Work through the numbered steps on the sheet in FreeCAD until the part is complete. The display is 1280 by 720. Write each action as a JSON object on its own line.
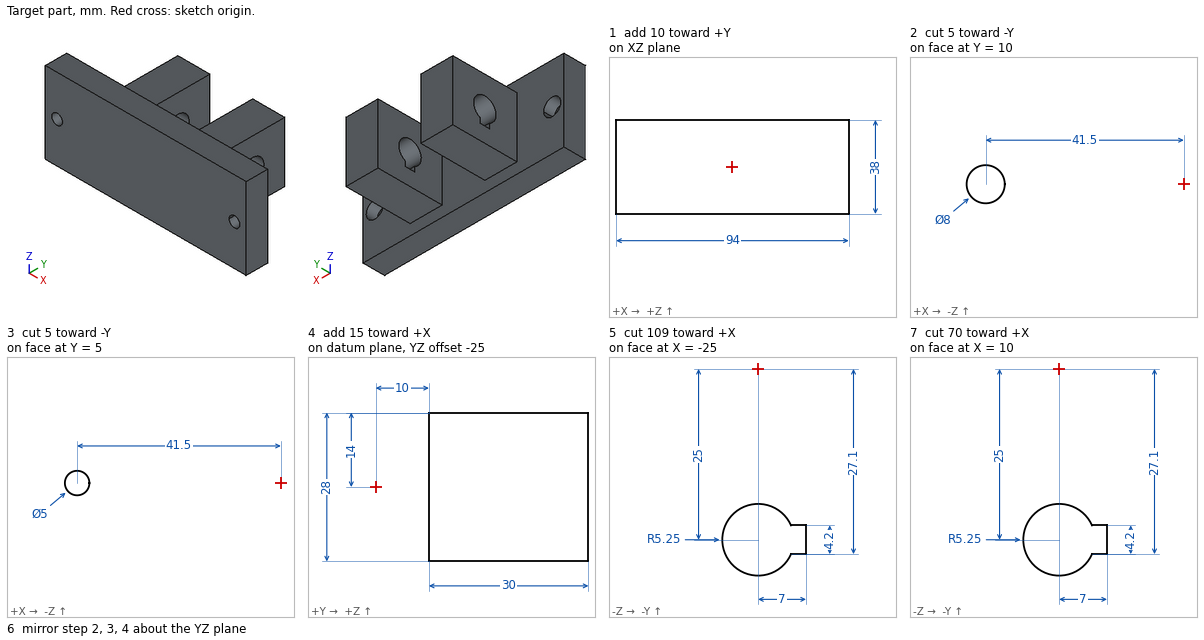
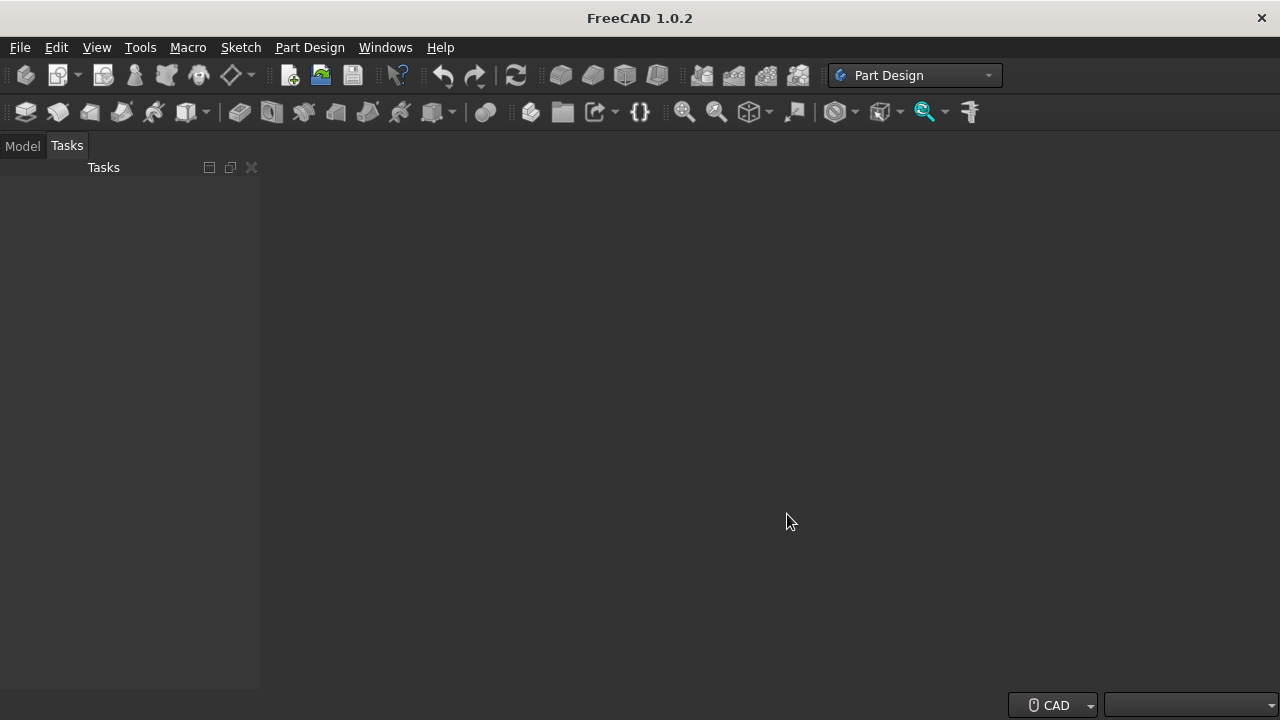
{"action": "left_click", "coordinate": [290, 76]}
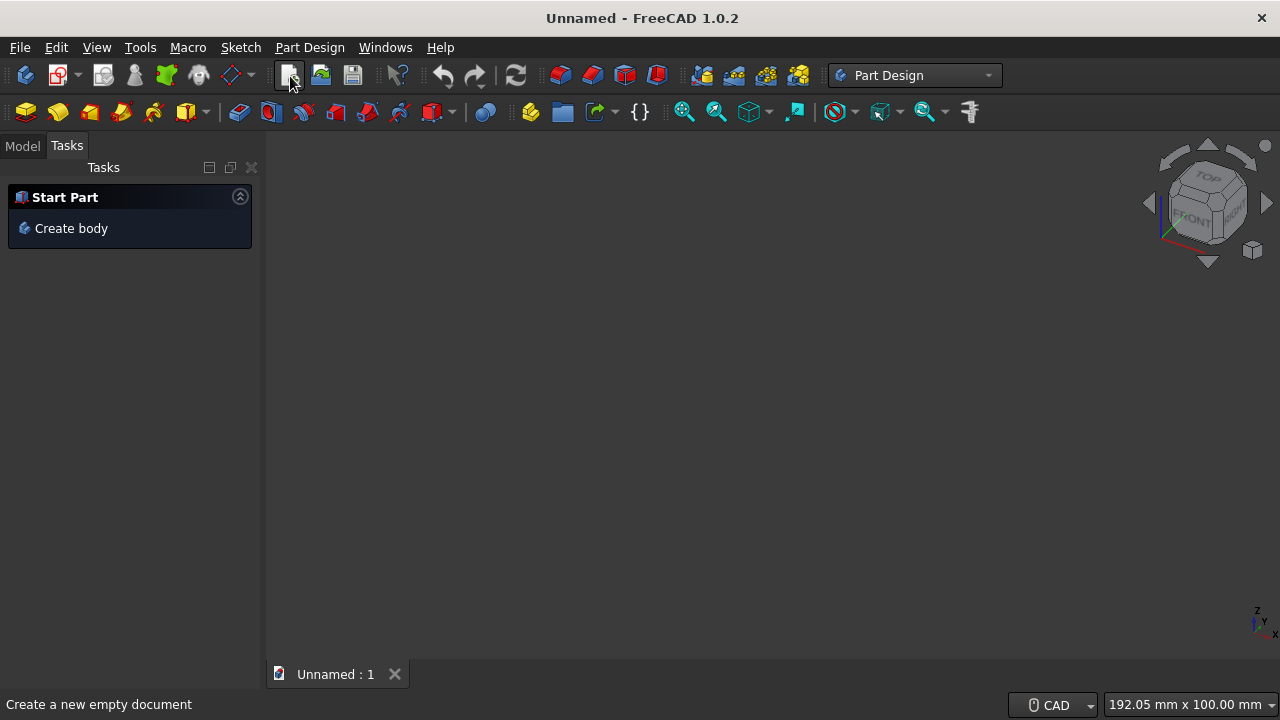
{"action": "left_click", "coordinate": [58, 76]}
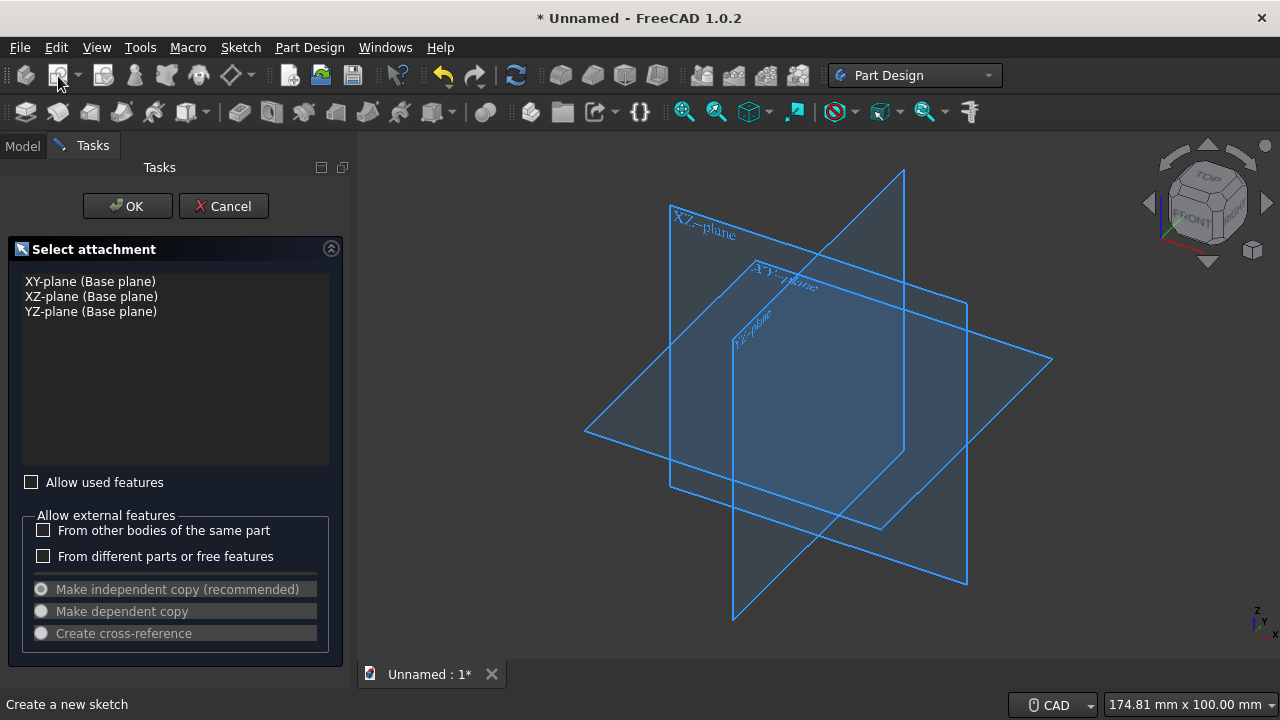
{"action": "left_click", "coordinate": [82, 296]}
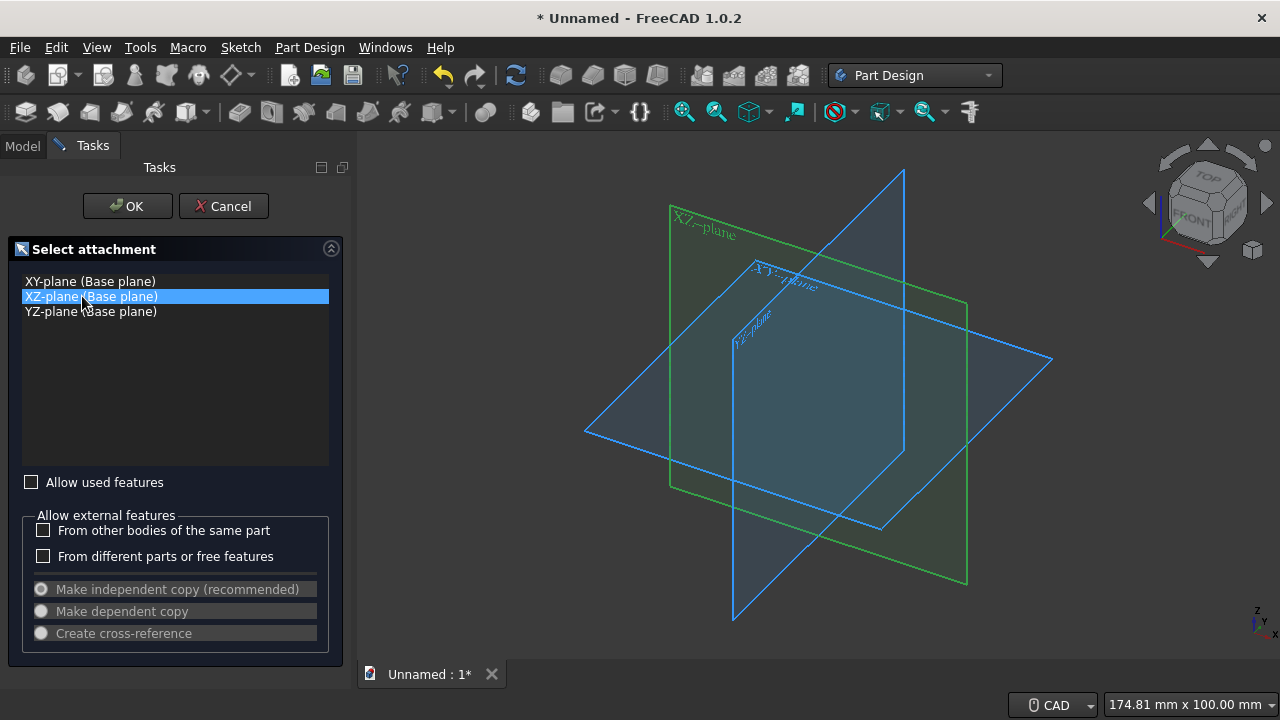
{"action": "left_click", "coordinate": [128, 206]}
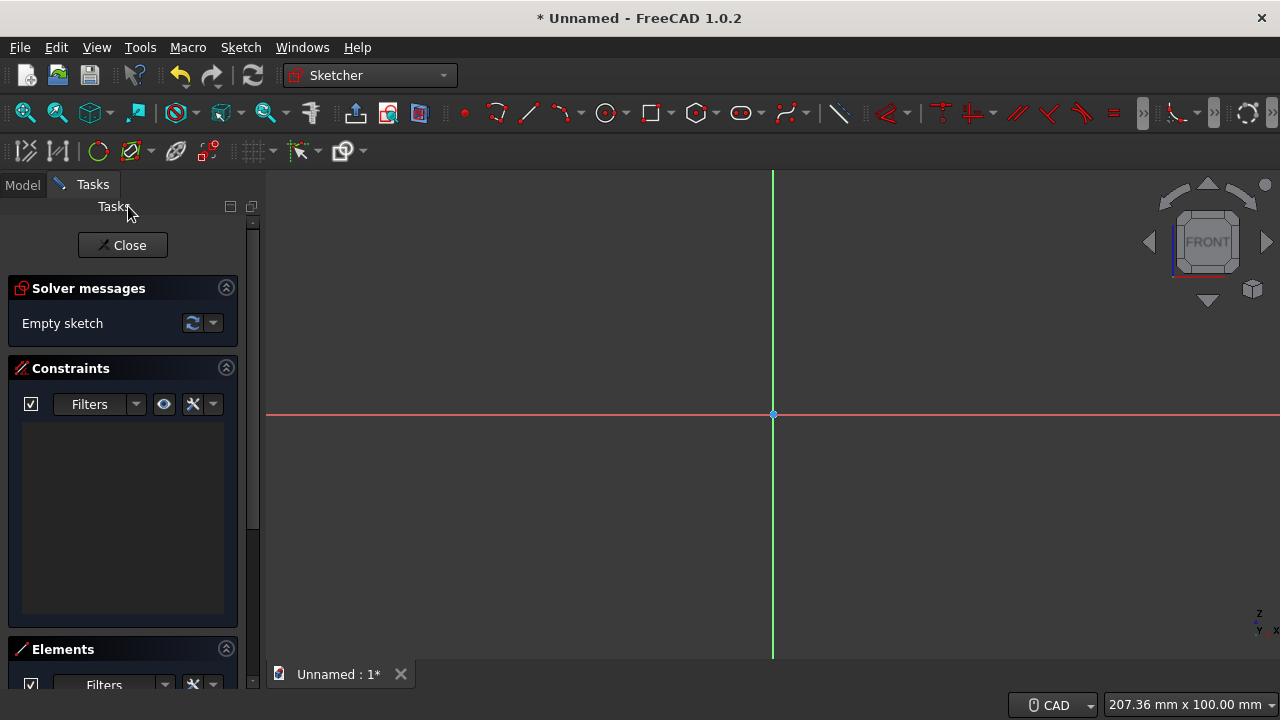
{"action": "left_click", "coordinate": [674, 114]}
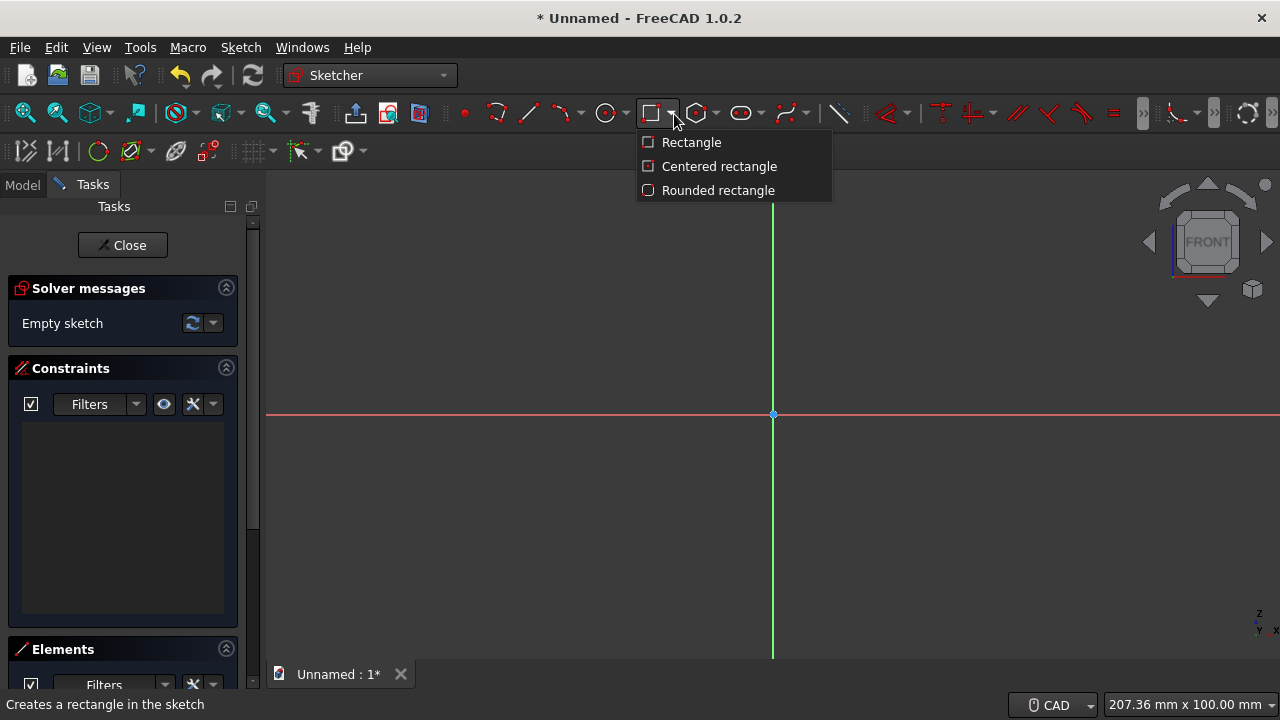
{"action": "left_click", "coordinate": [734, 166]}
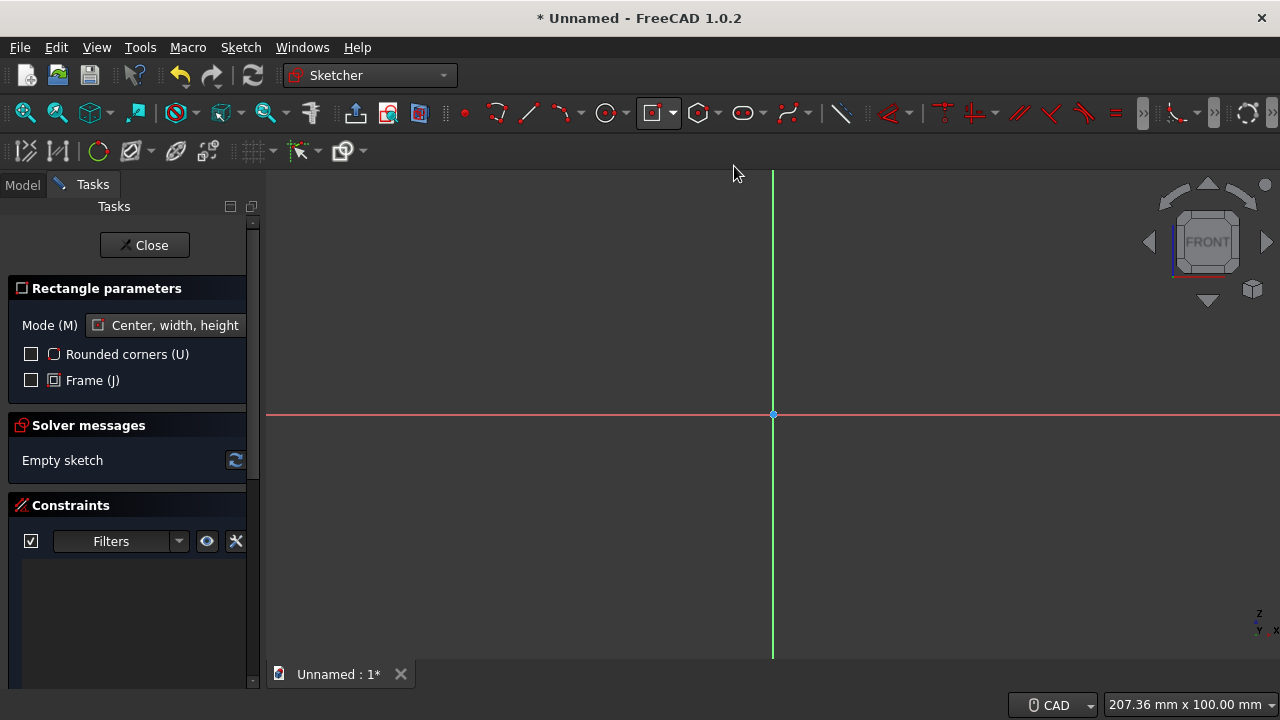
{"action": "left_click", "coordinate": [773, 414]}
{"action": "left_click", "coordinate": [1003, 322]}
{"action": "key", "text": "Escape"}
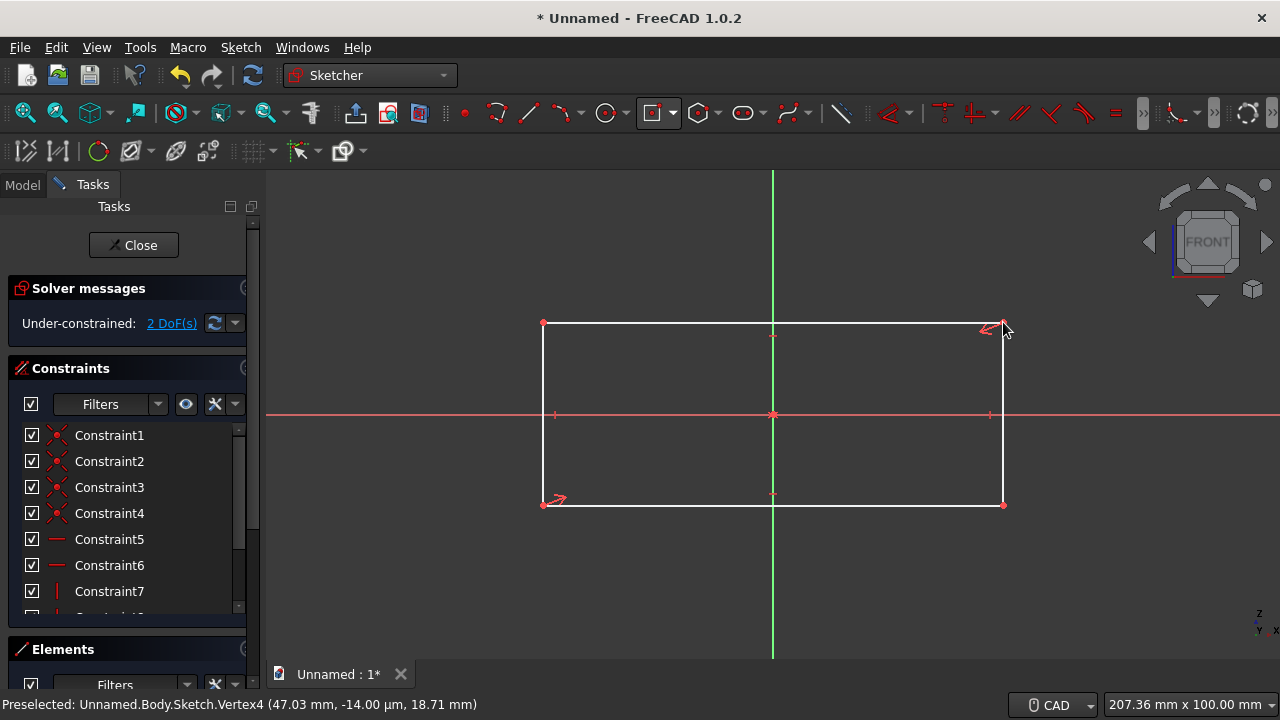
{"action": "left_click", "coordinate": [888, 114]}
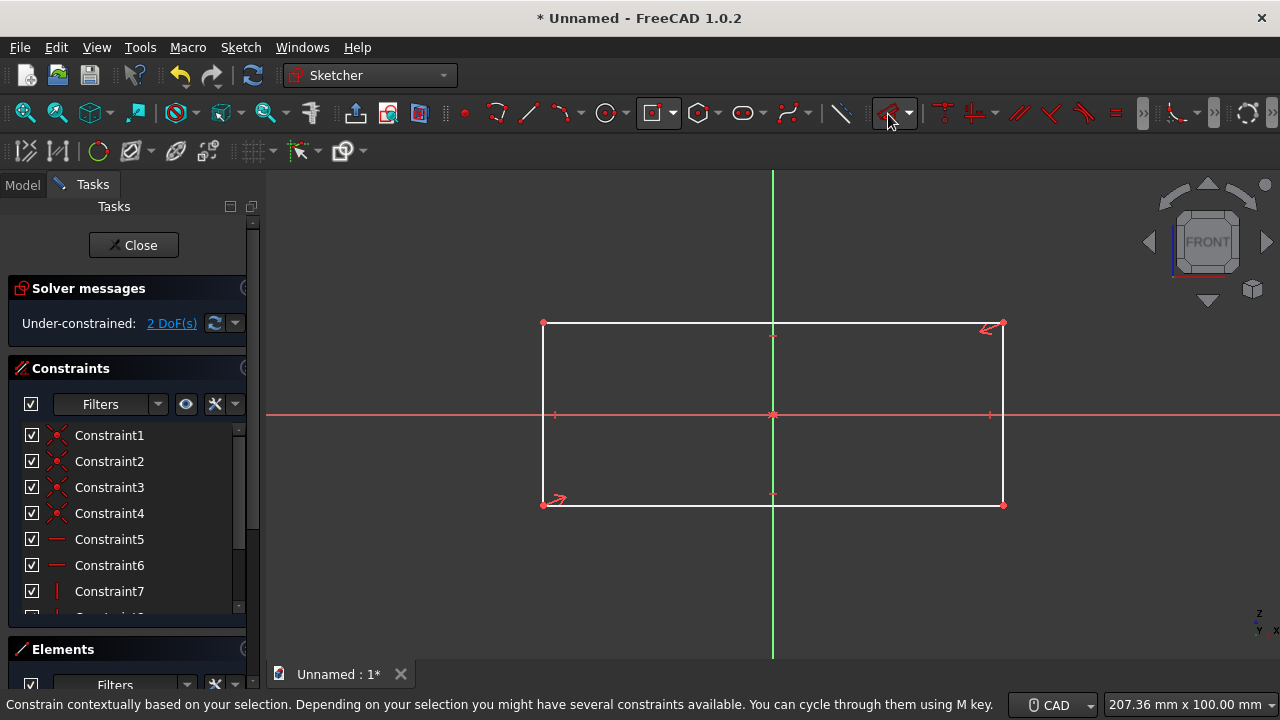
{"action": "left_click", "coordinate": [681, 506]}
{"action": "left_click", "coordinate": [667, 540]}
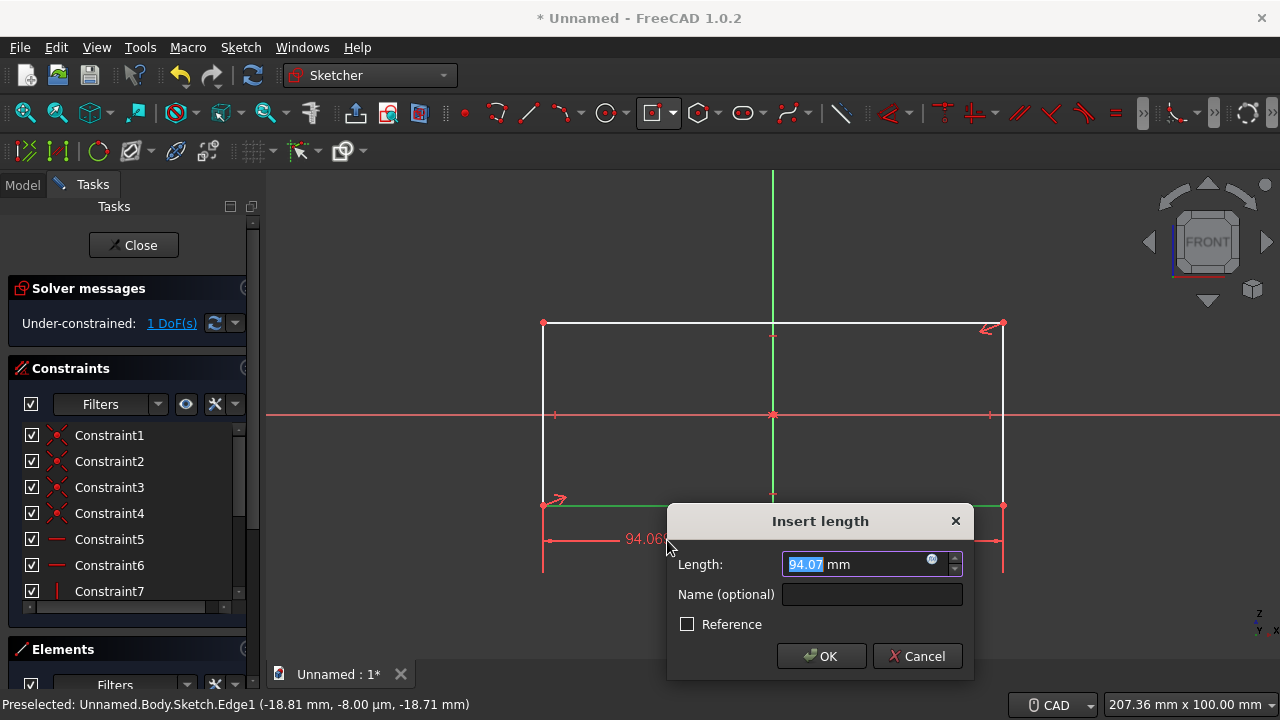
{"action": "type", "text": "94"}
{"action": "key", "text": "Return"}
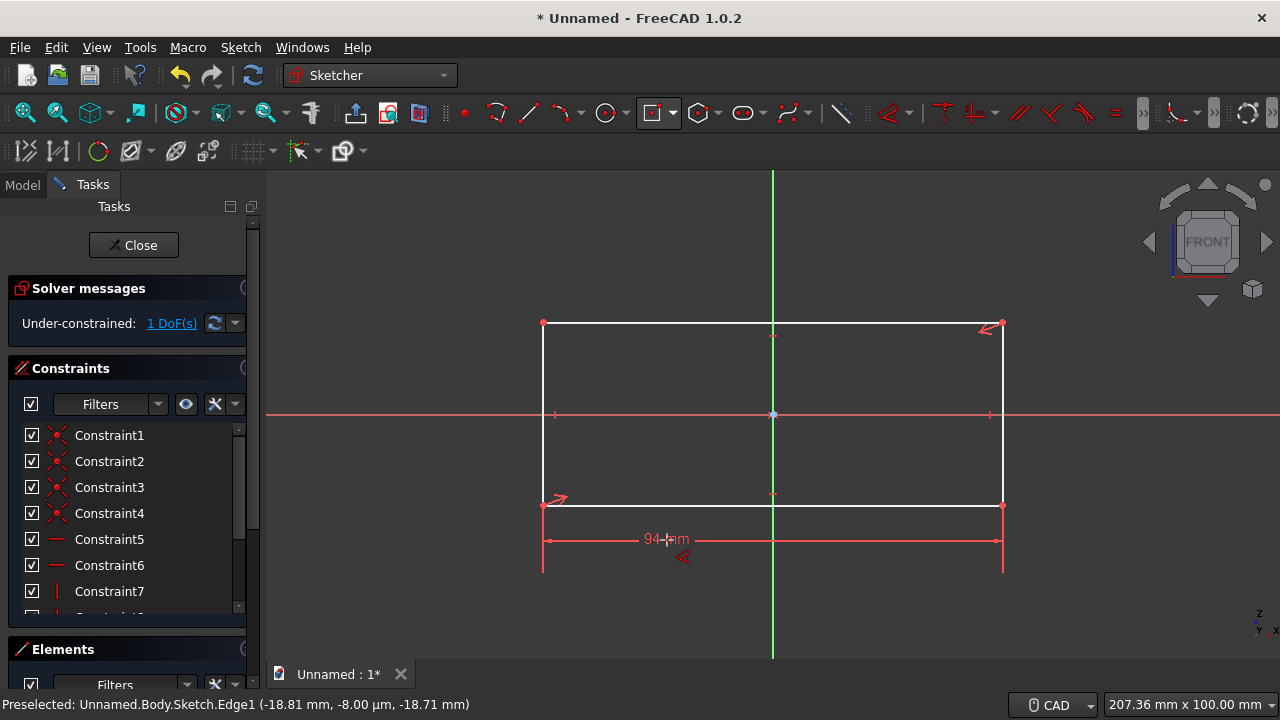
{"action": "left_click", "coordinate": [1003, 451]}
{"action": "left_click", "coordinate": [1037, 372]}